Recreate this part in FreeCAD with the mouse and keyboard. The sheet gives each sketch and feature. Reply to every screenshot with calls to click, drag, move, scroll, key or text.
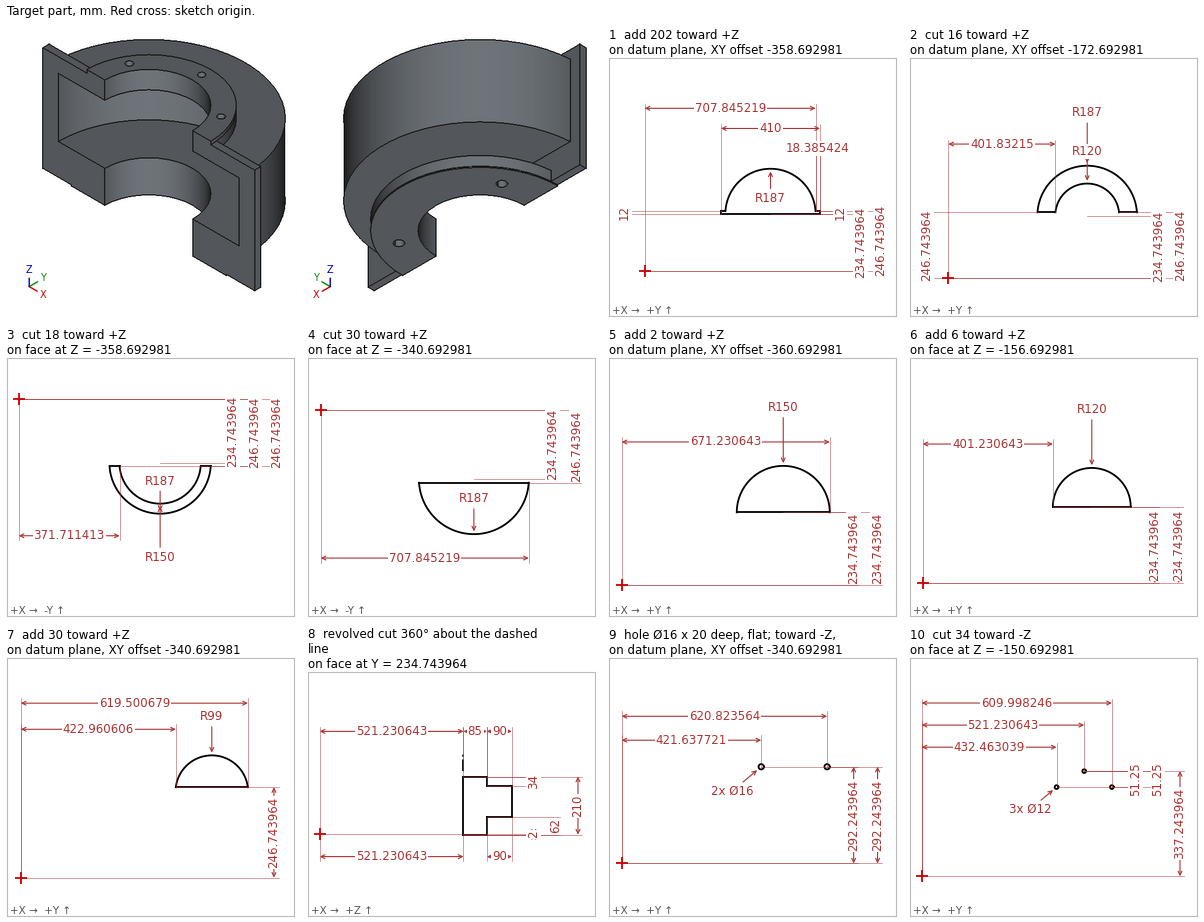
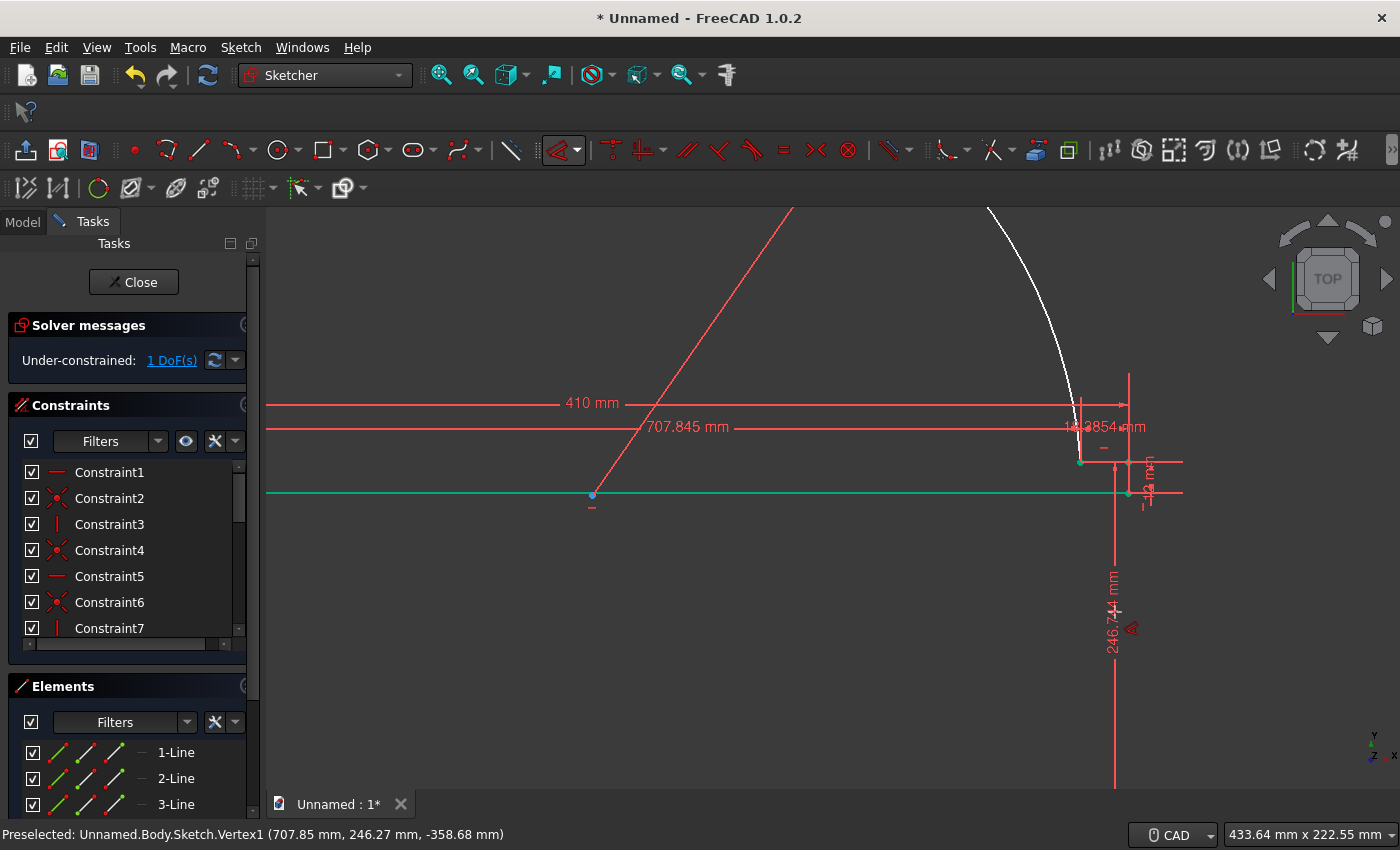
click(593, 496)
click(627, 628)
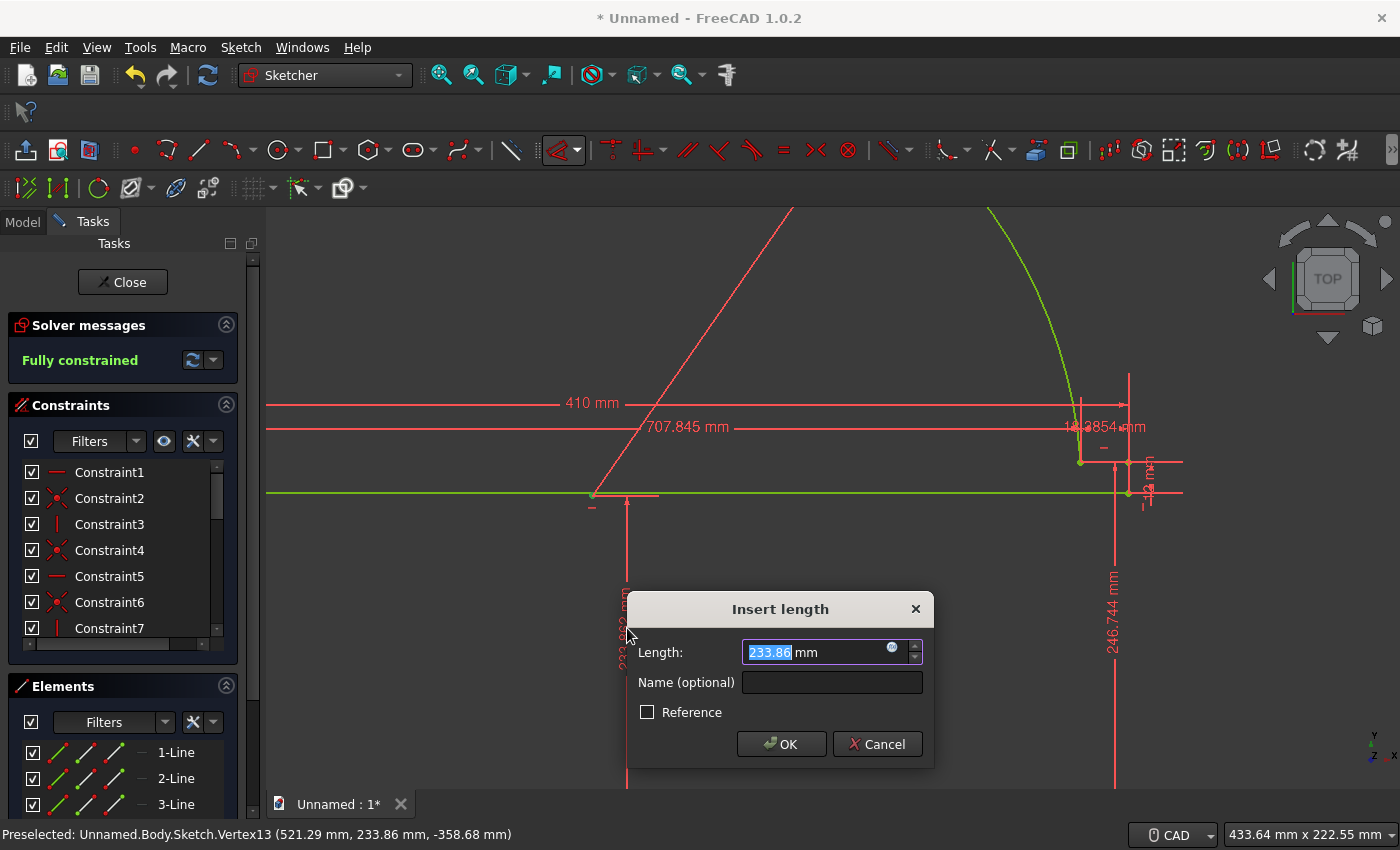
text(234.743964)
key(Return)
key(Escape)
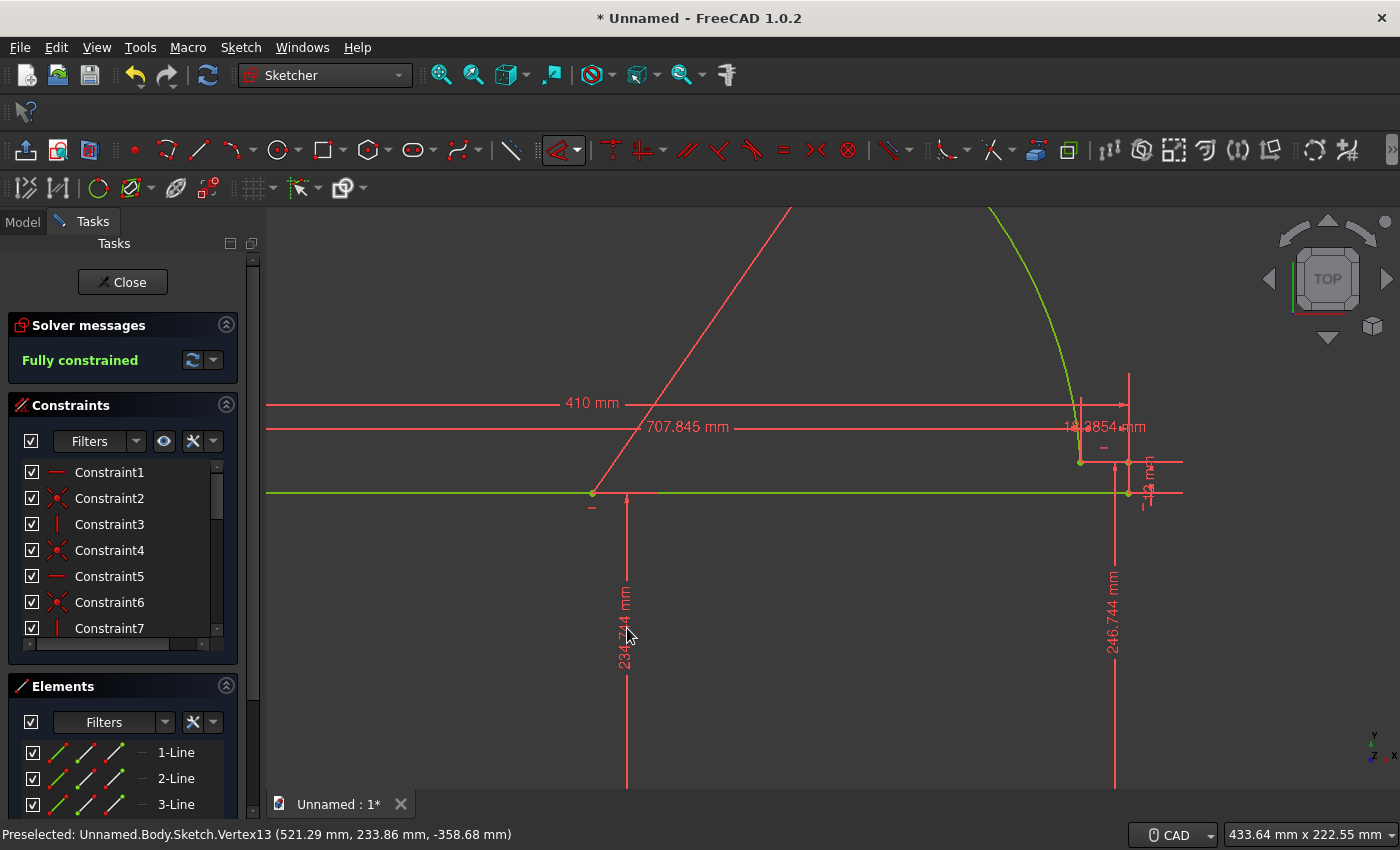
click(123, 282)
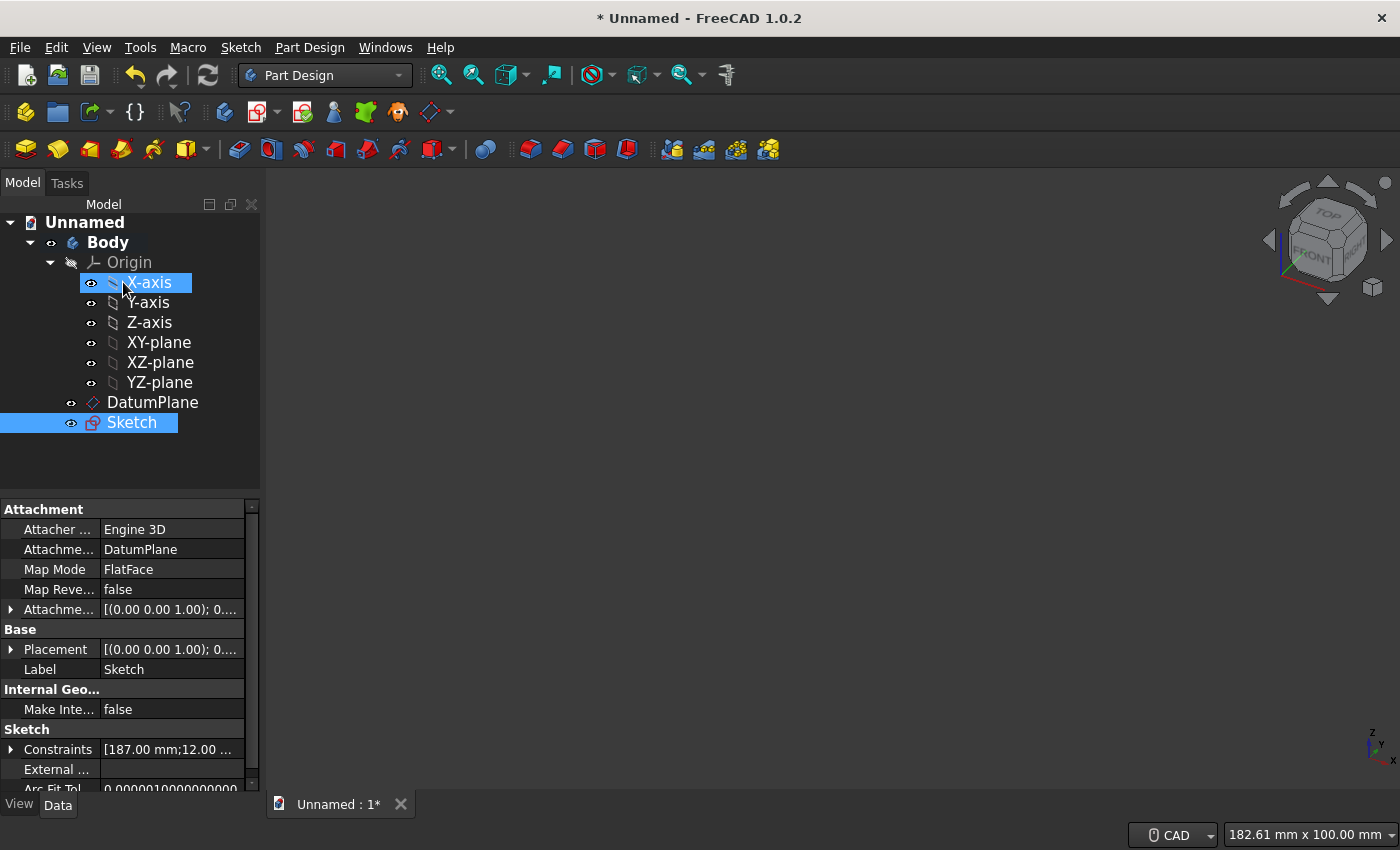
click(26, 150)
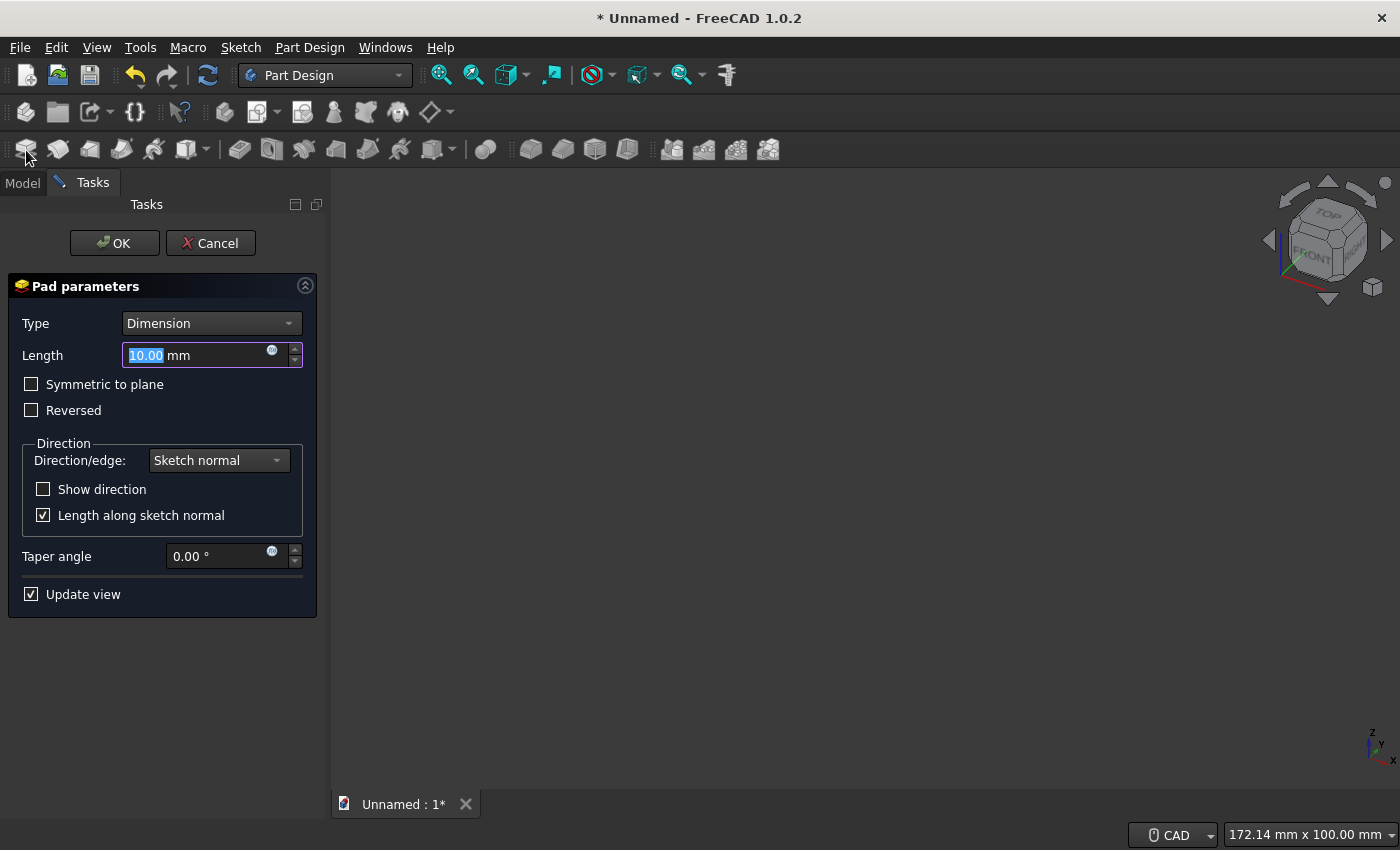
text(202)
key(Tab)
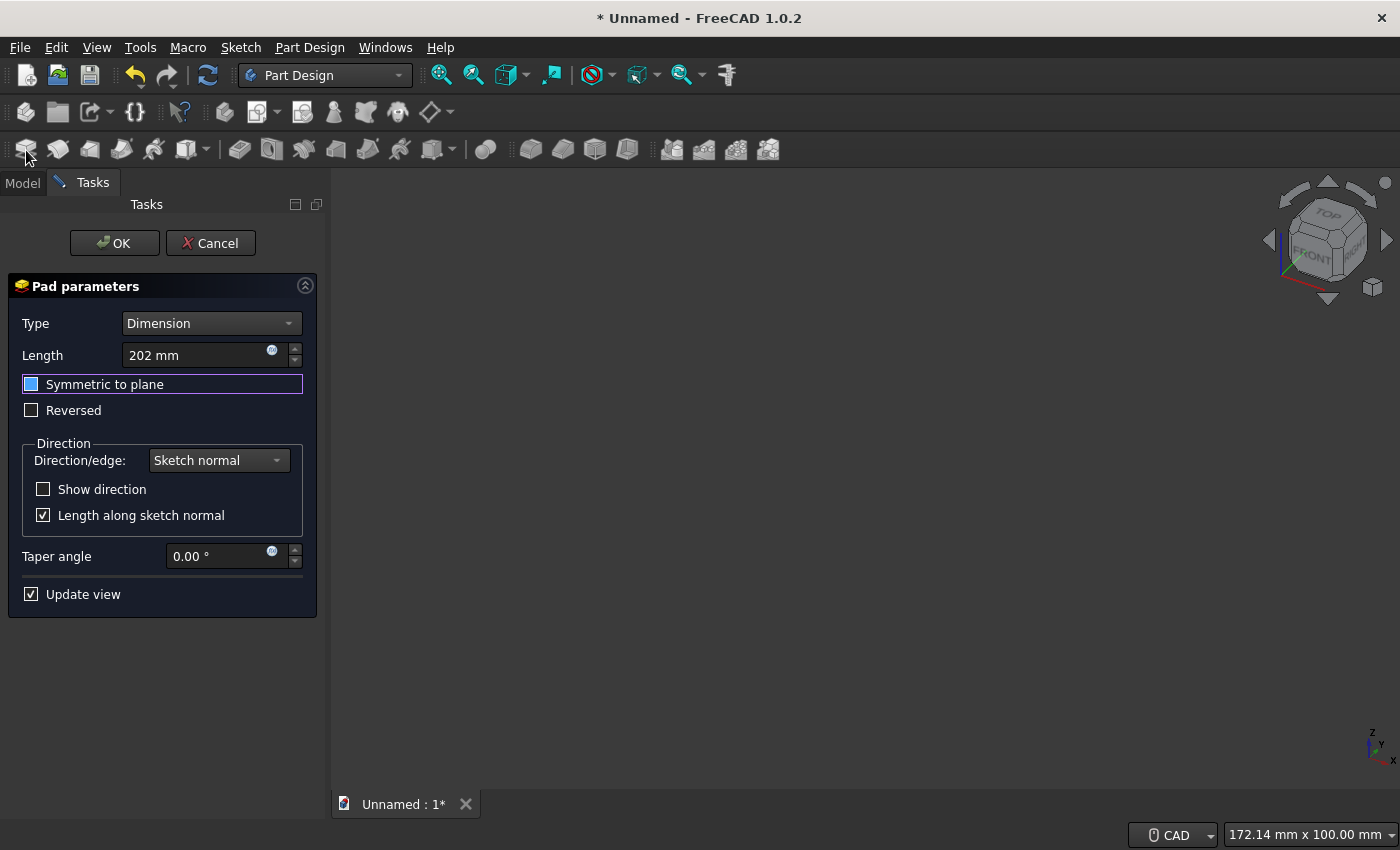
click(115, 243)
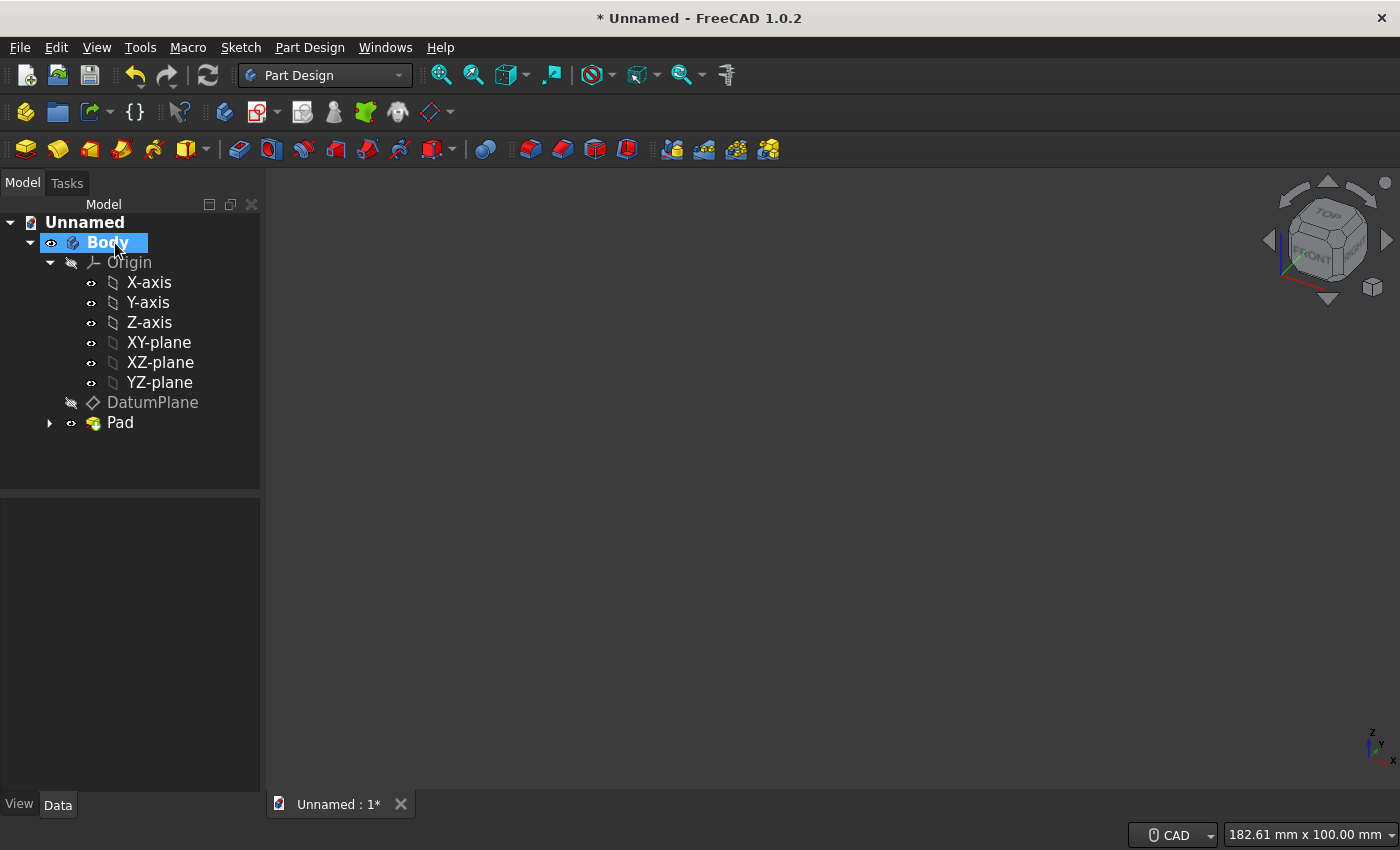
click(442, 76)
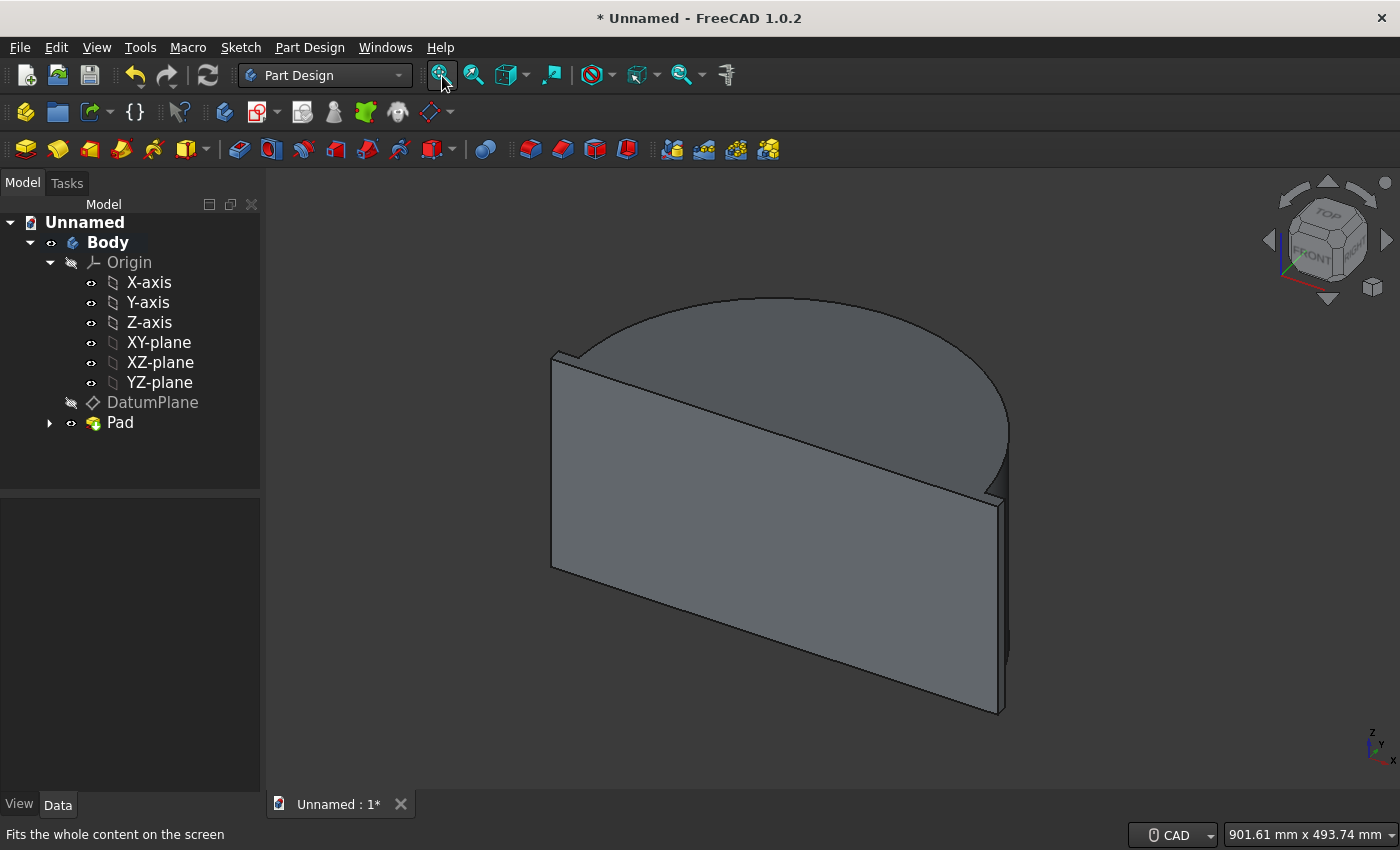
click(136, 343)